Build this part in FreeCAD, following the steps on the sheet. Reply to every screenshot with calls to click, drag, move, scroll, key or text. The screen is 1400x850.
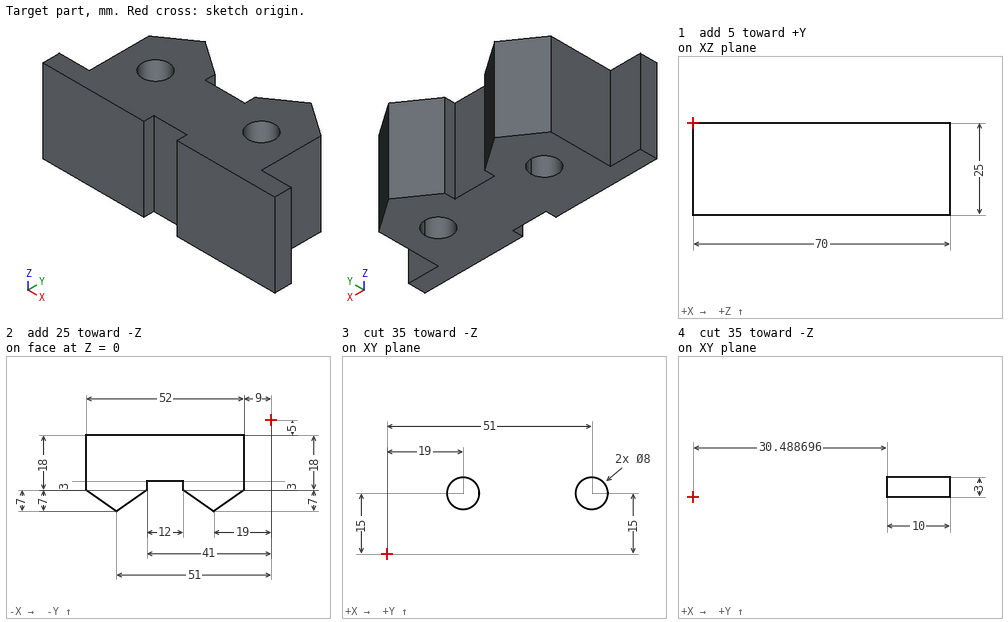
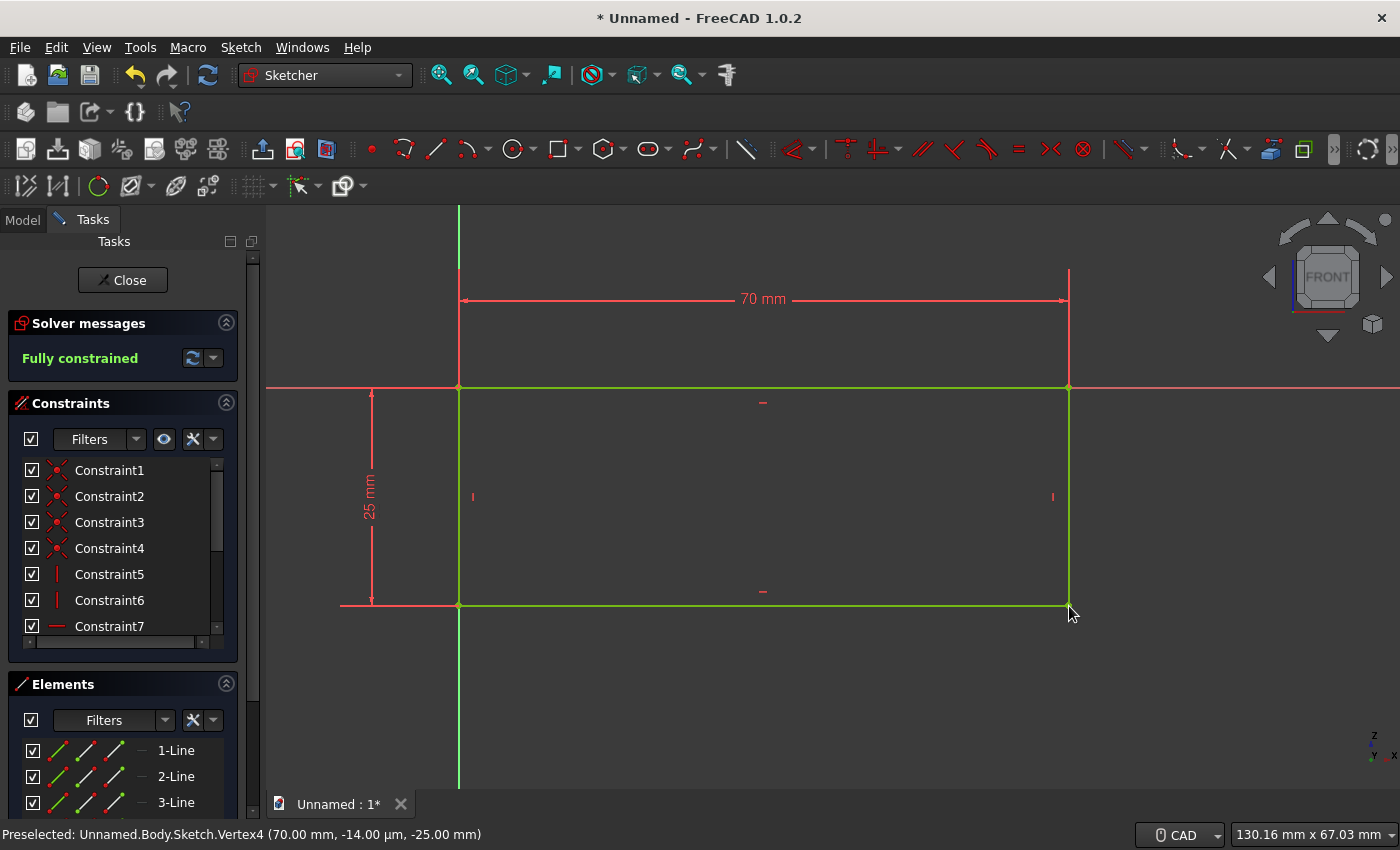
click(123, 280)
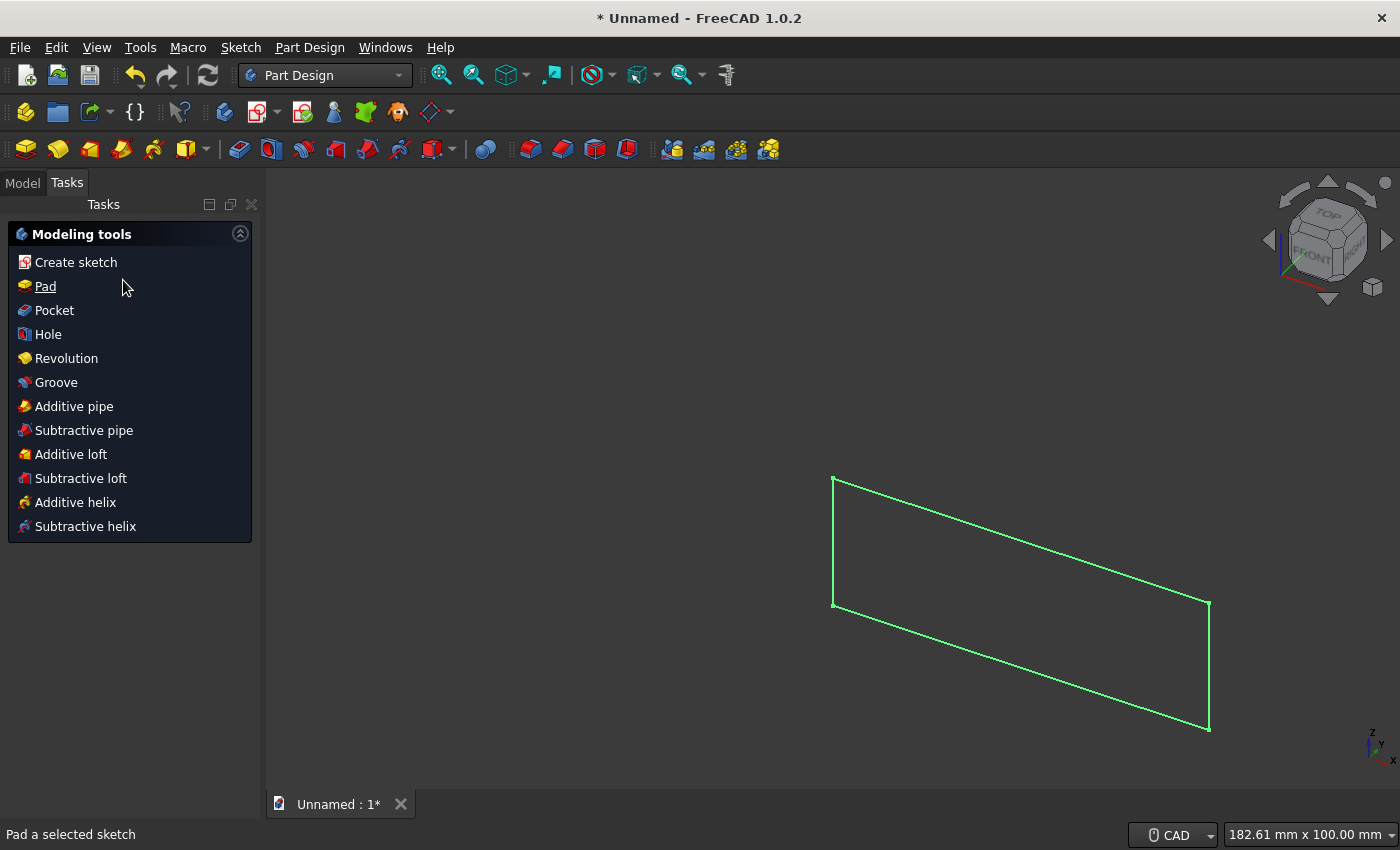
click(26, 150)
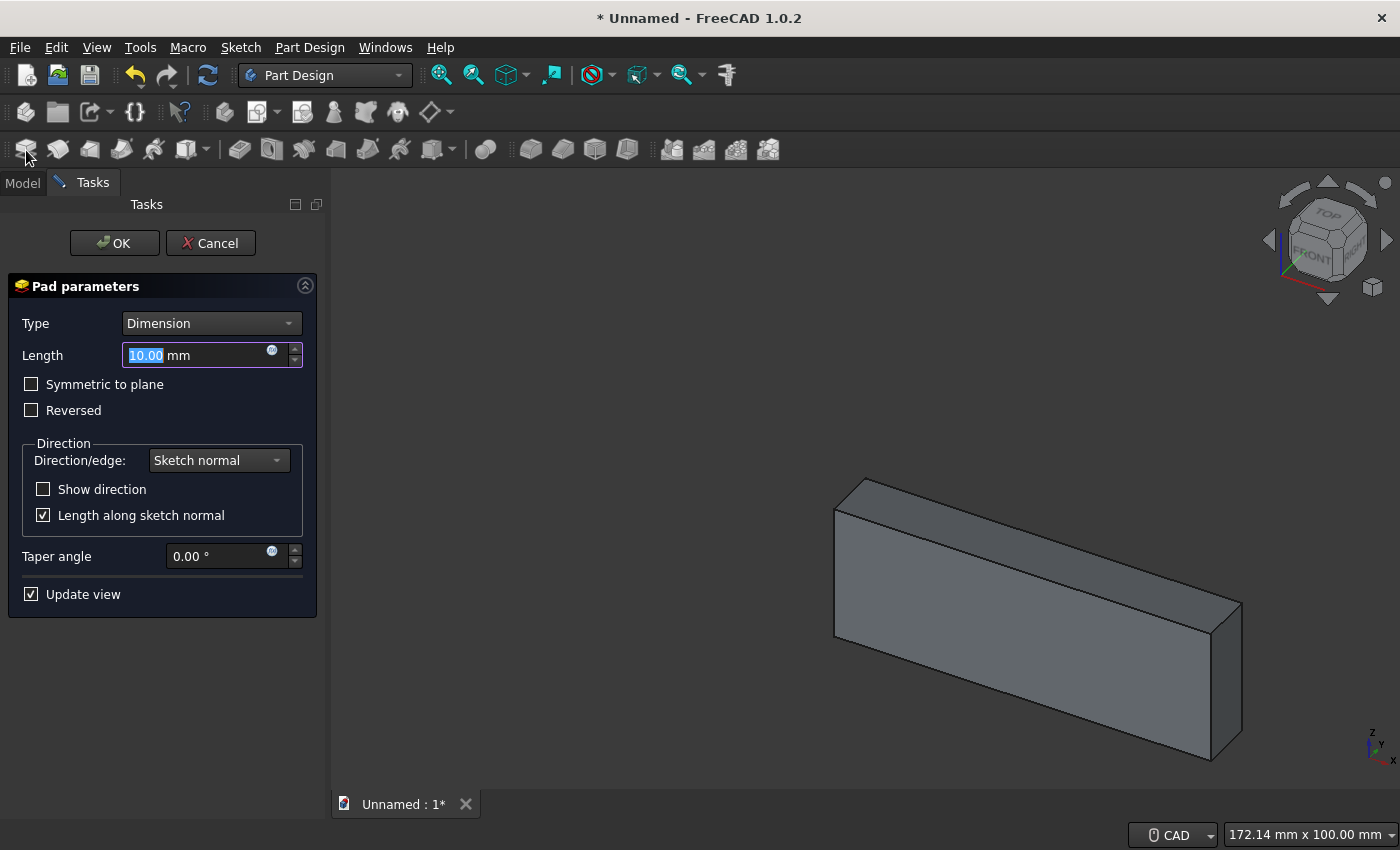
text(5)
key(Tab)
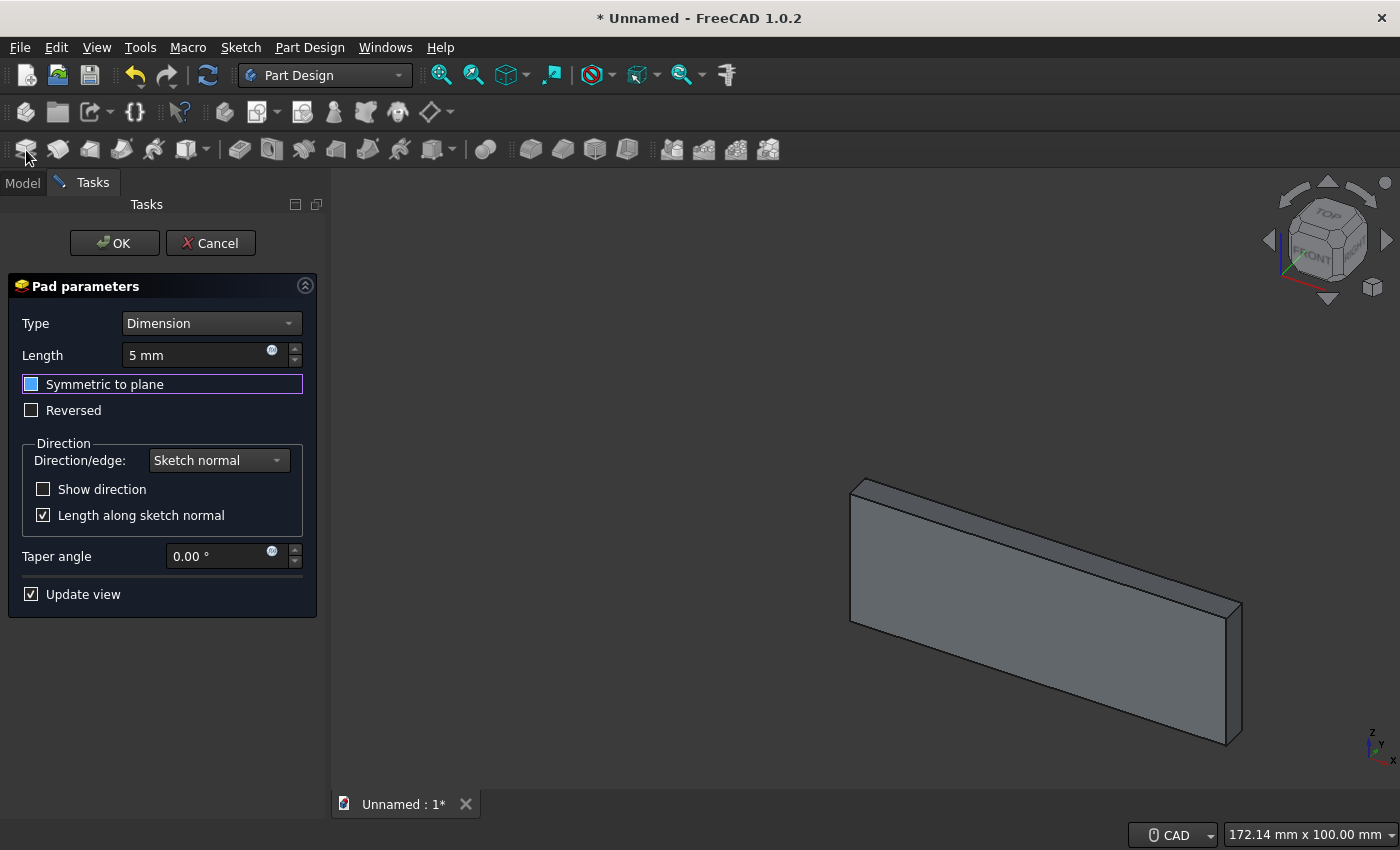
click(30, 410)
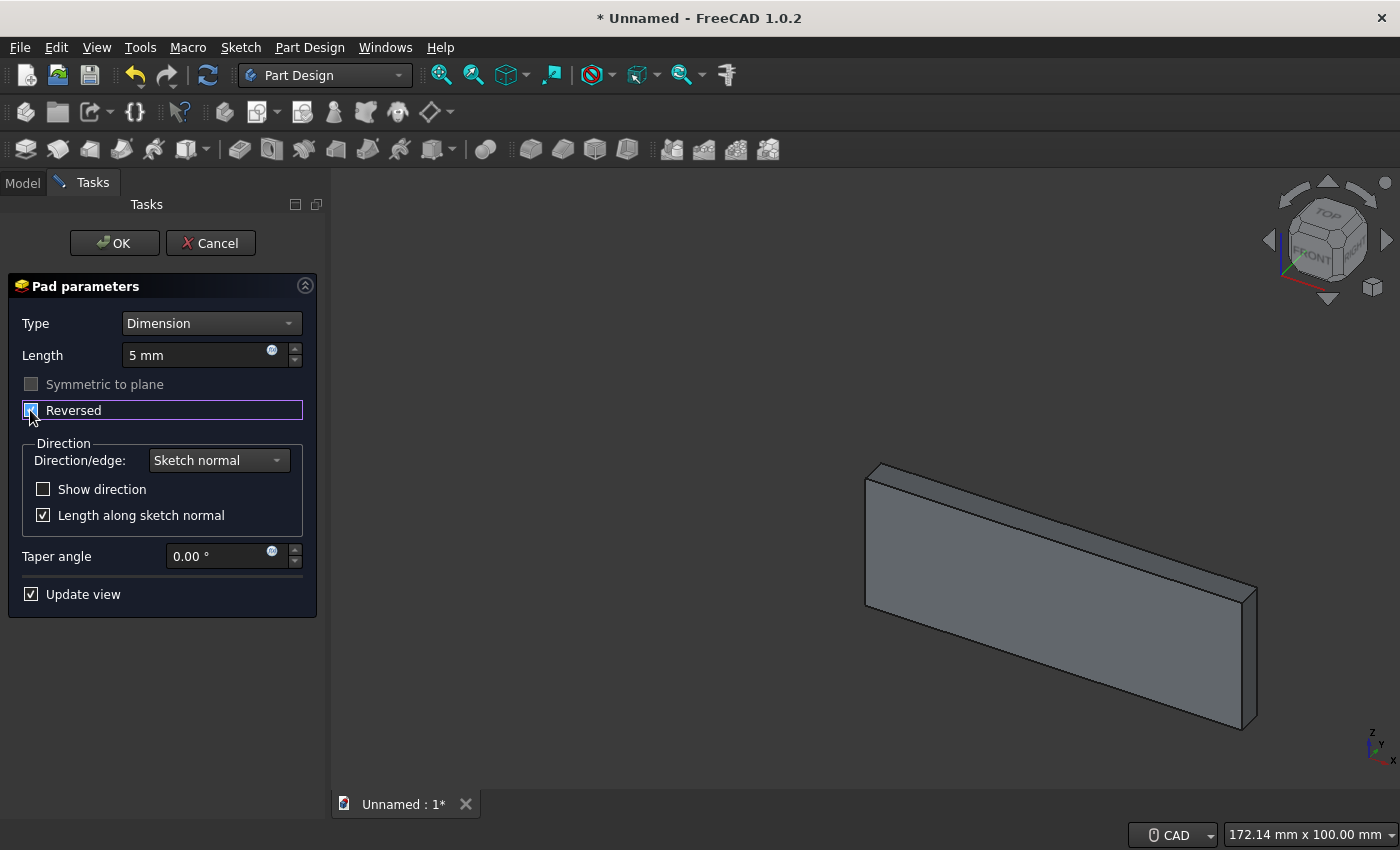
click(115, 243)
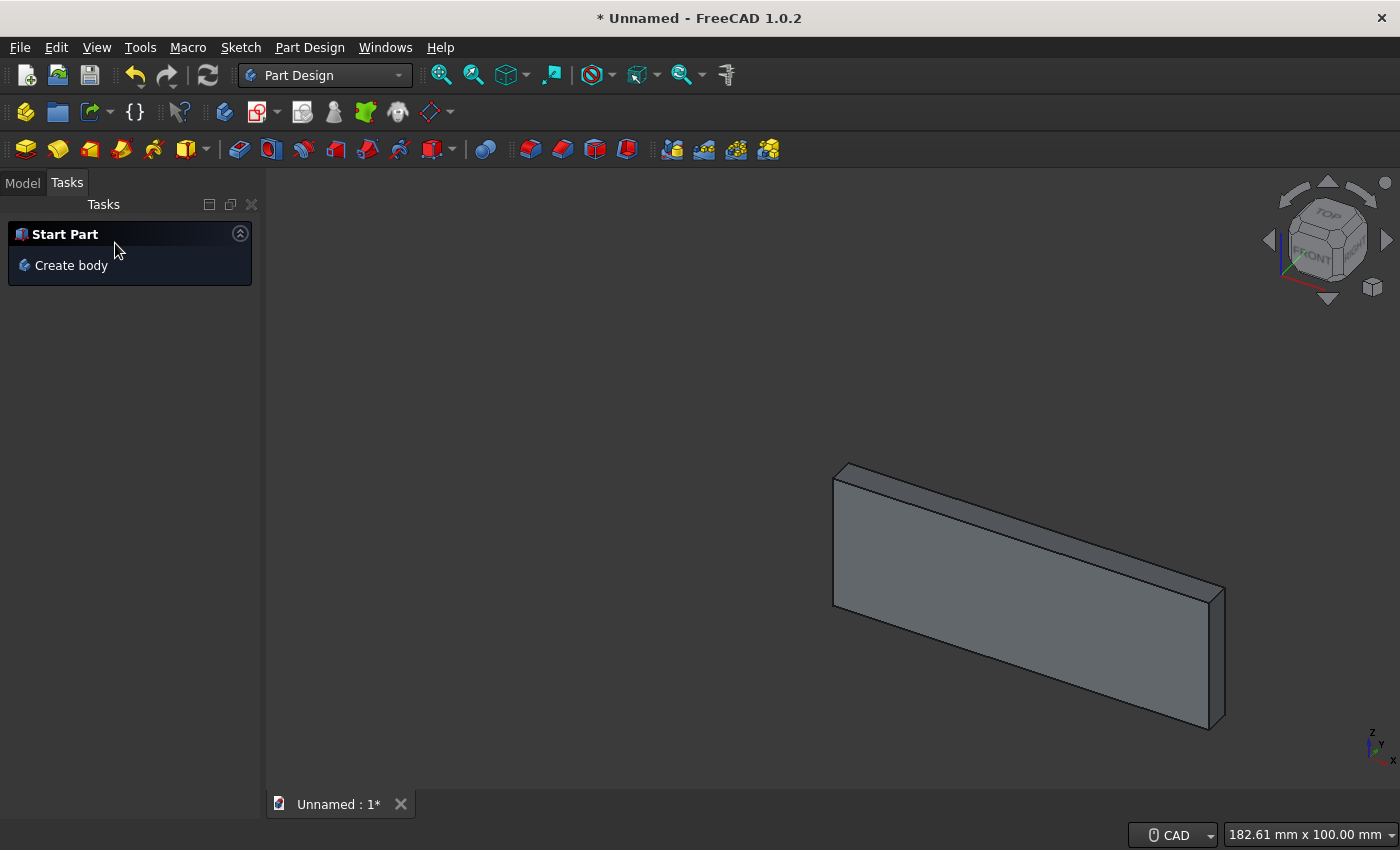
key(v)
key(f)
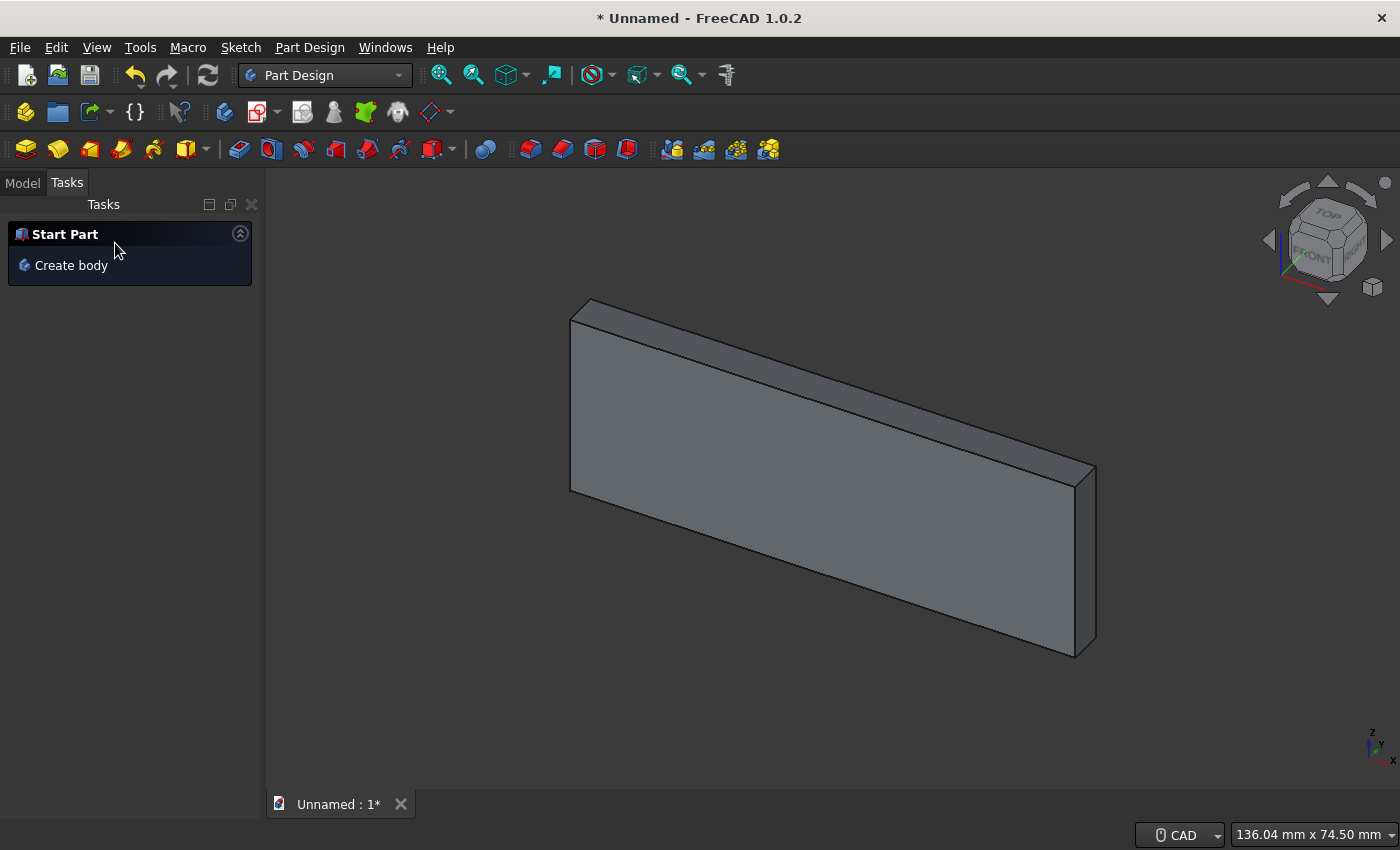
click(1050, 464)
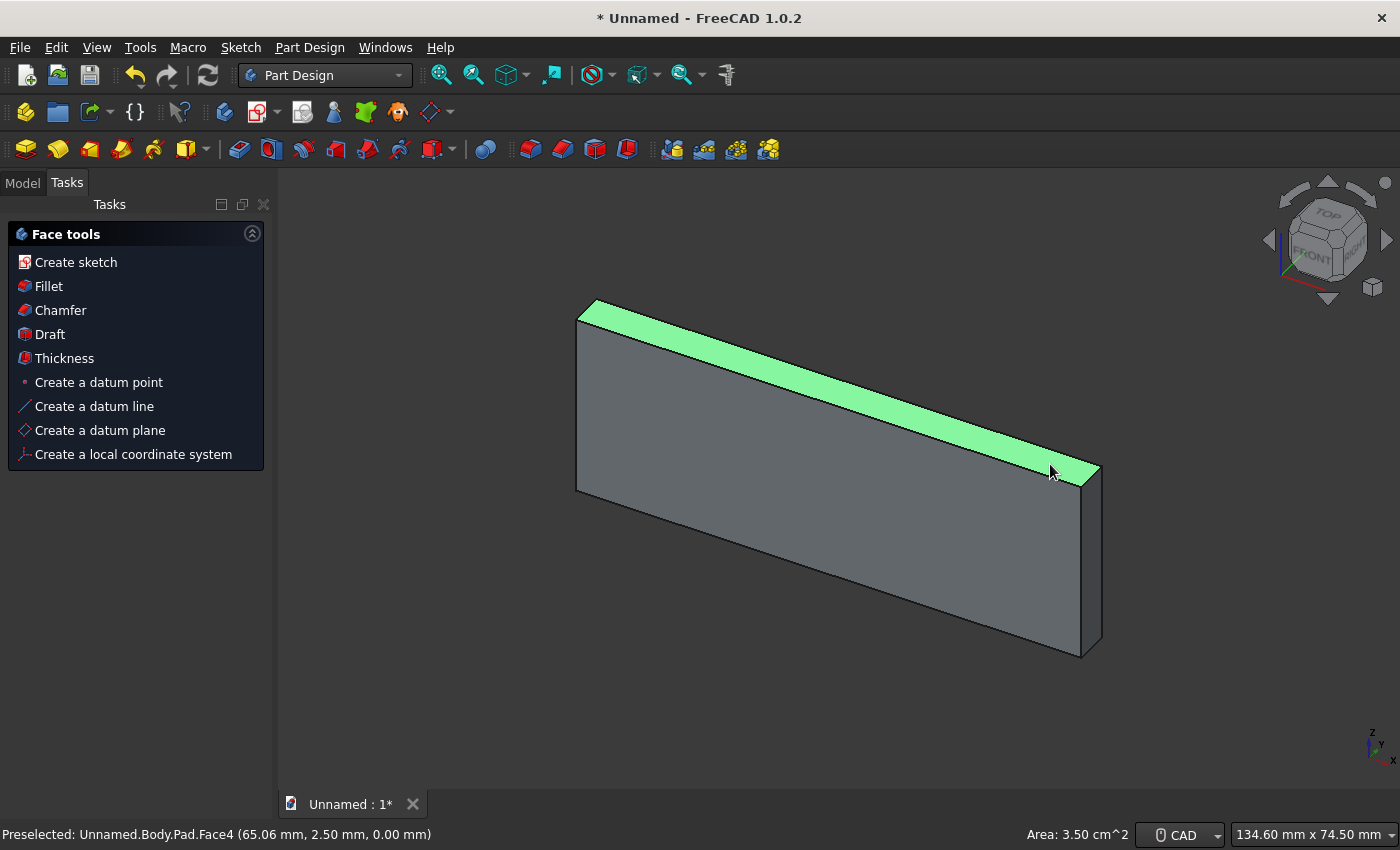
click(258, 112)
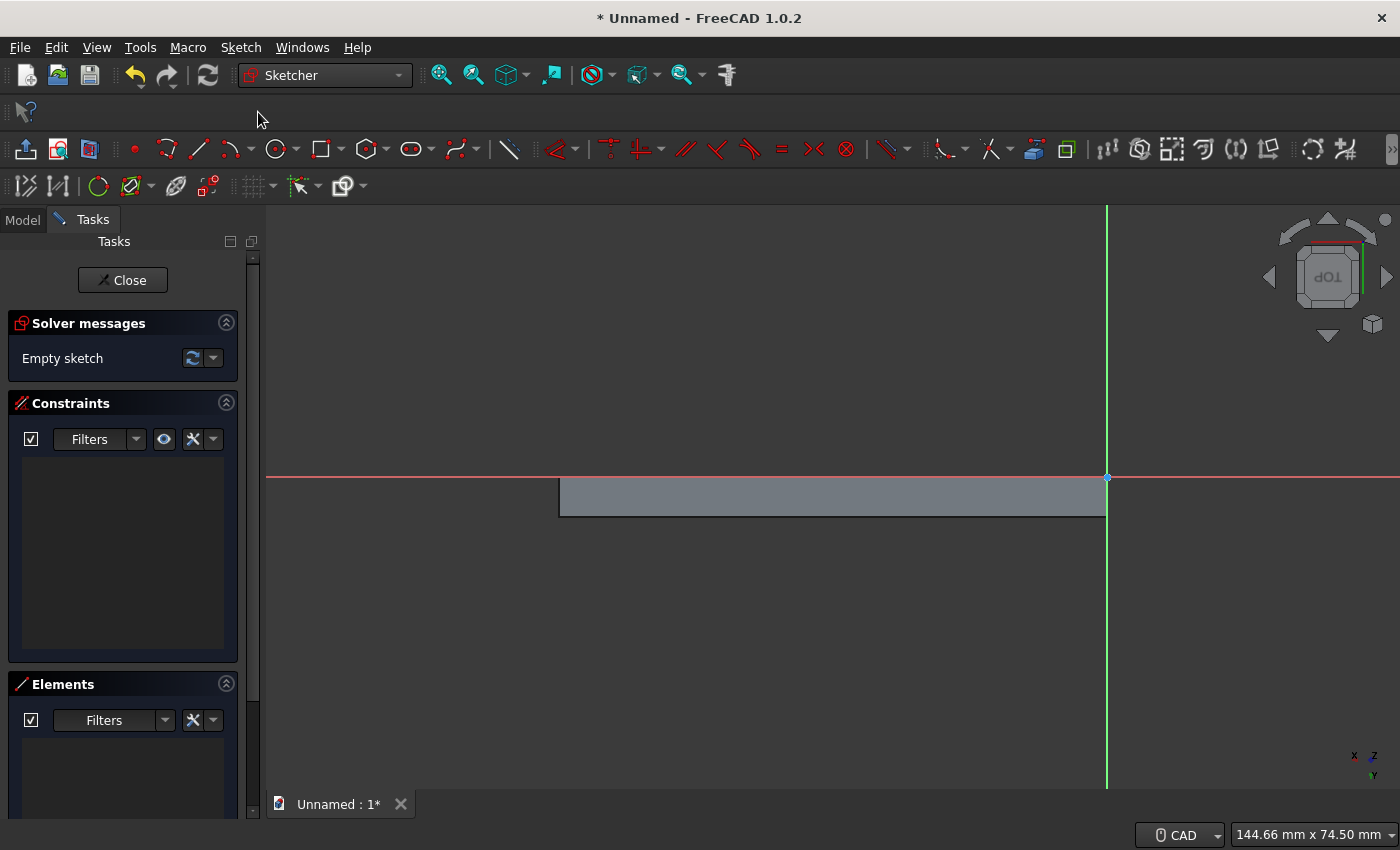
scroll(1079, 761, up, 2)